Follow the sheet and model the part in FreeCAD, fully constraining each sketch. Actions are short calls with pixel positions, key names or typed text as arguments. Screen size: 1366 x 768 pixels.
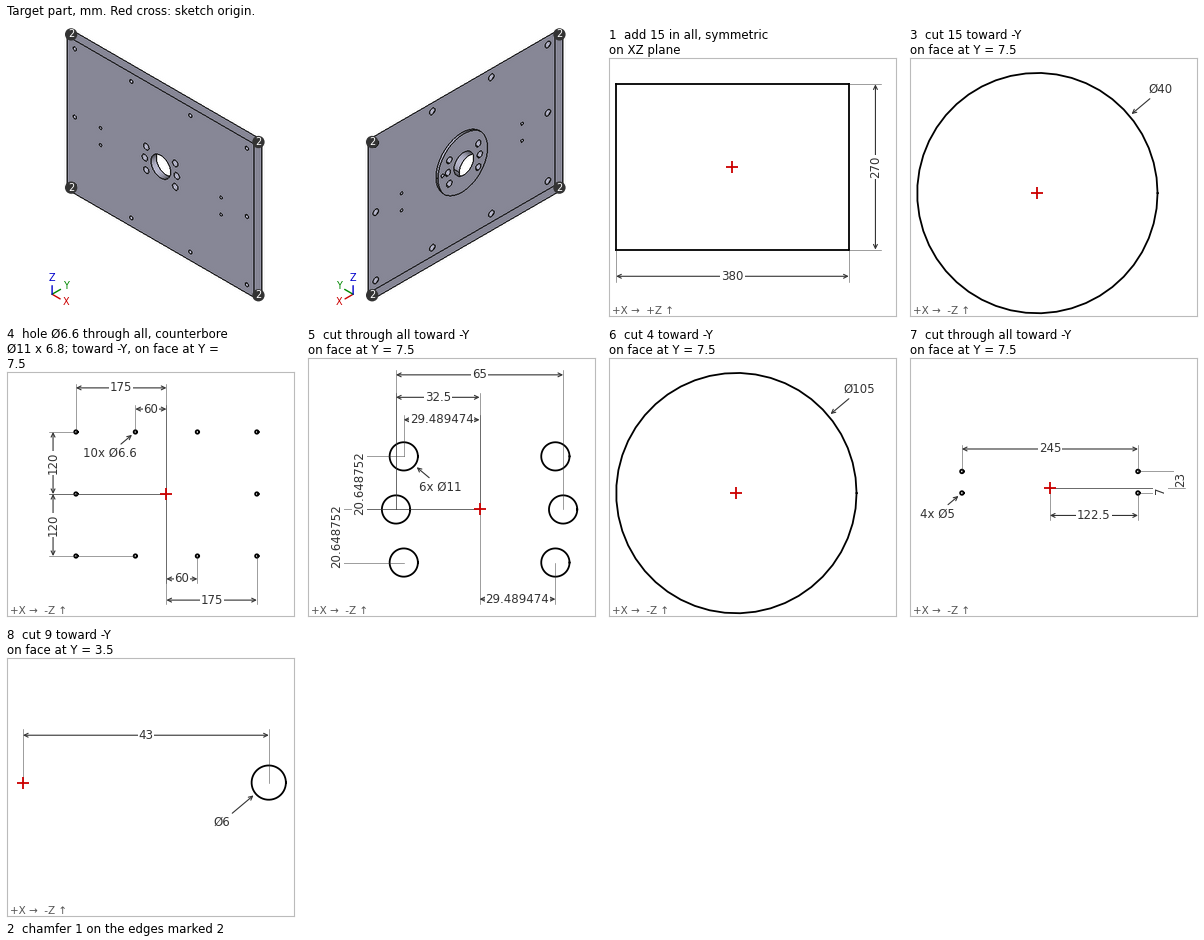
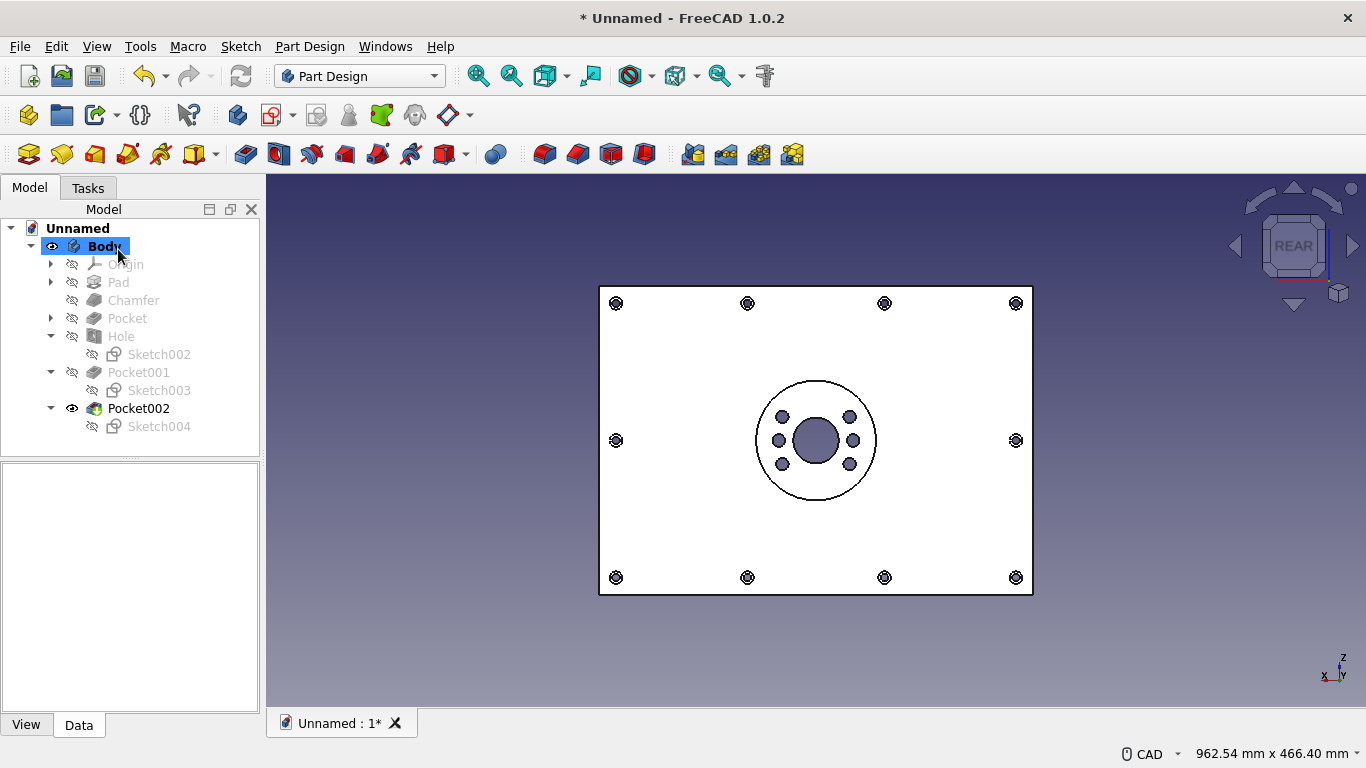
click(940, 395)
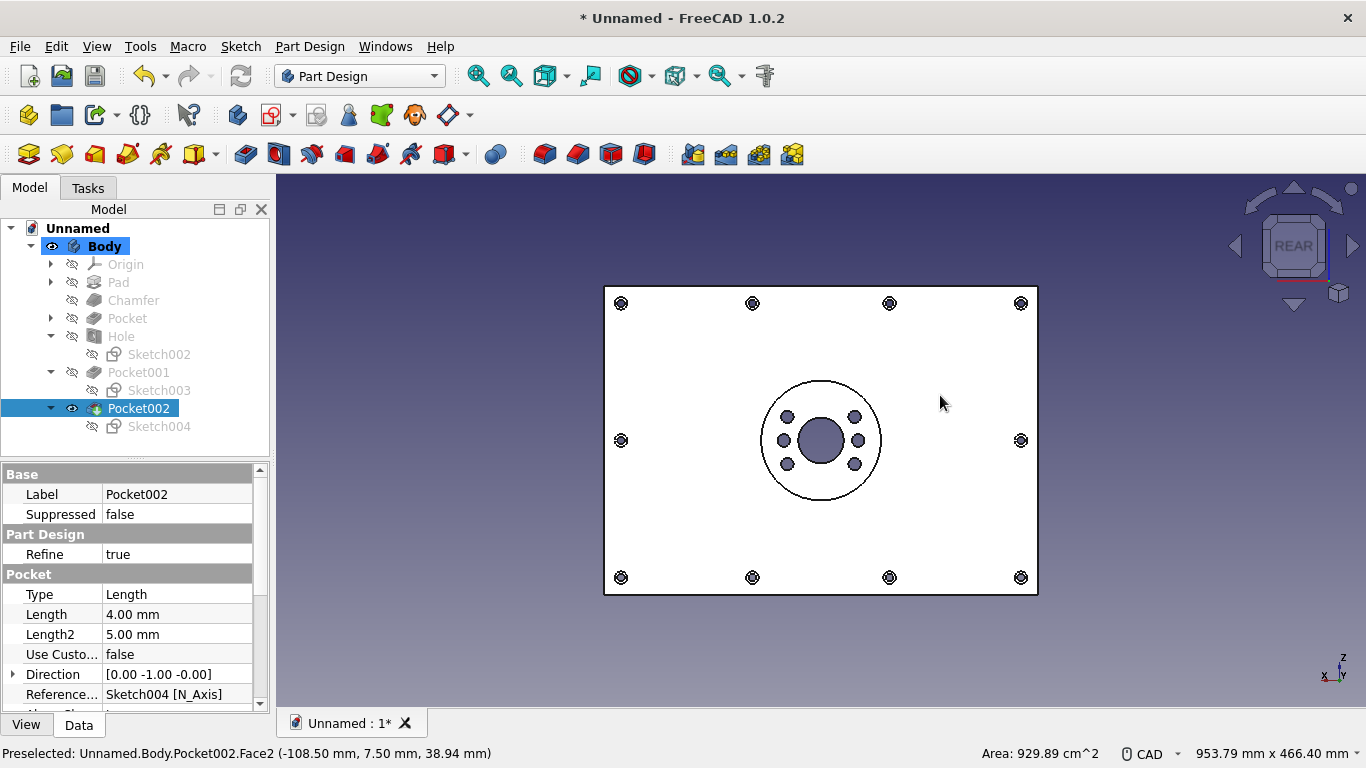
click(270, 116)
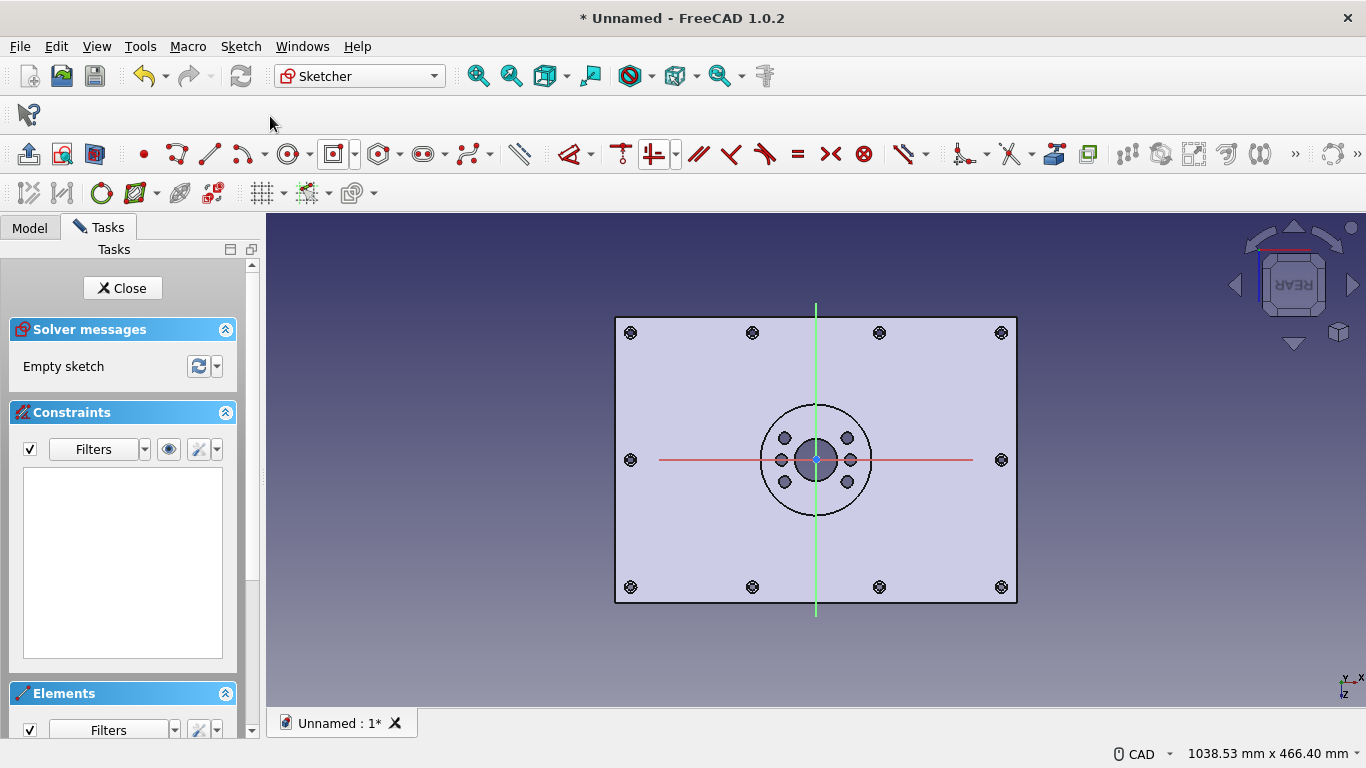
scroll(872, 445, up, 4)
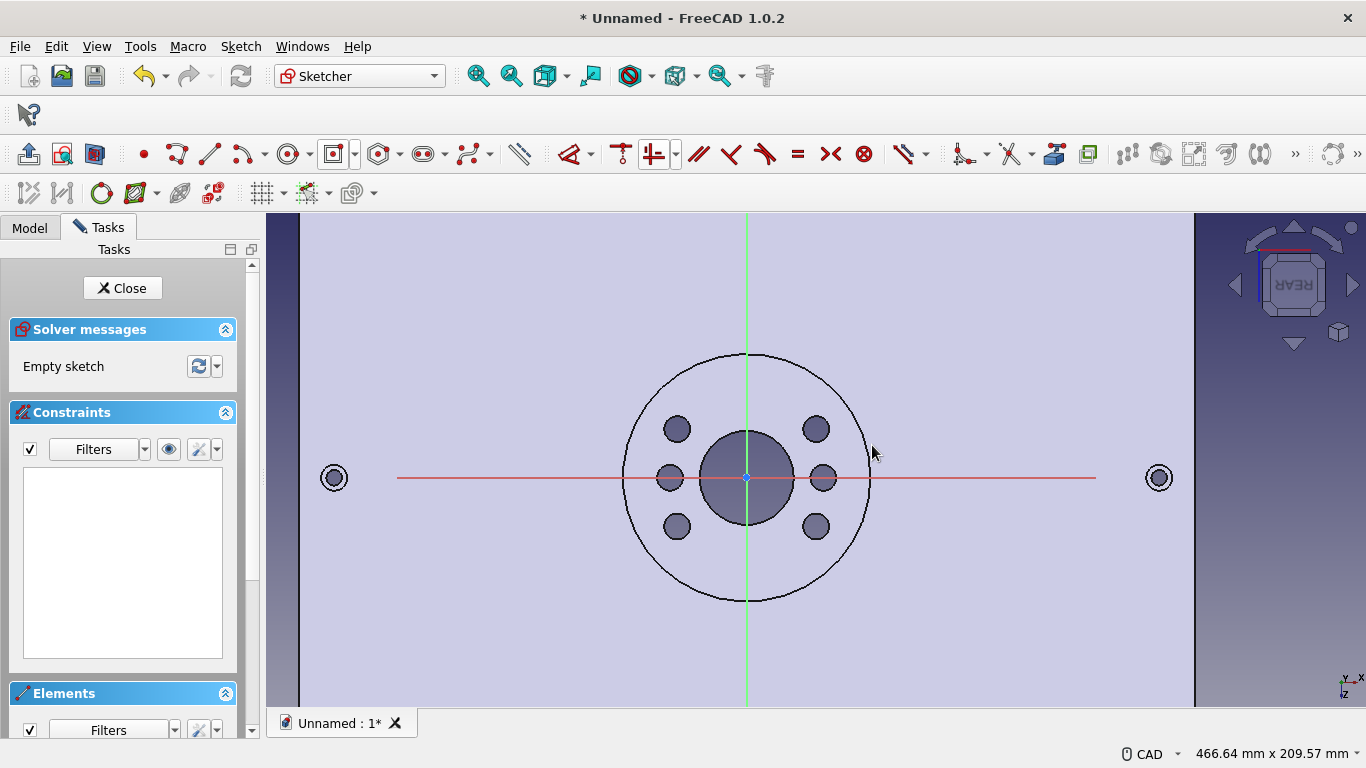
click(288, 154)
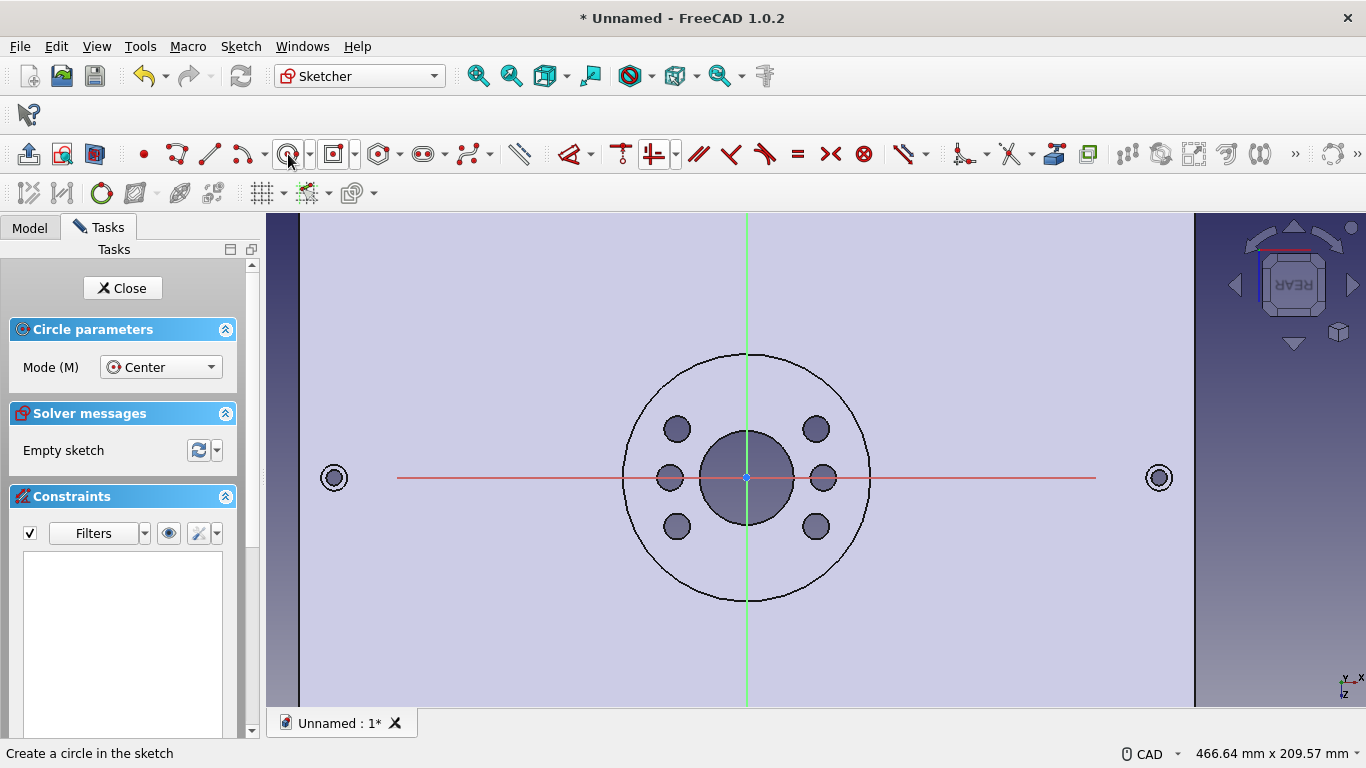
scroll(1035, 494, up, 7)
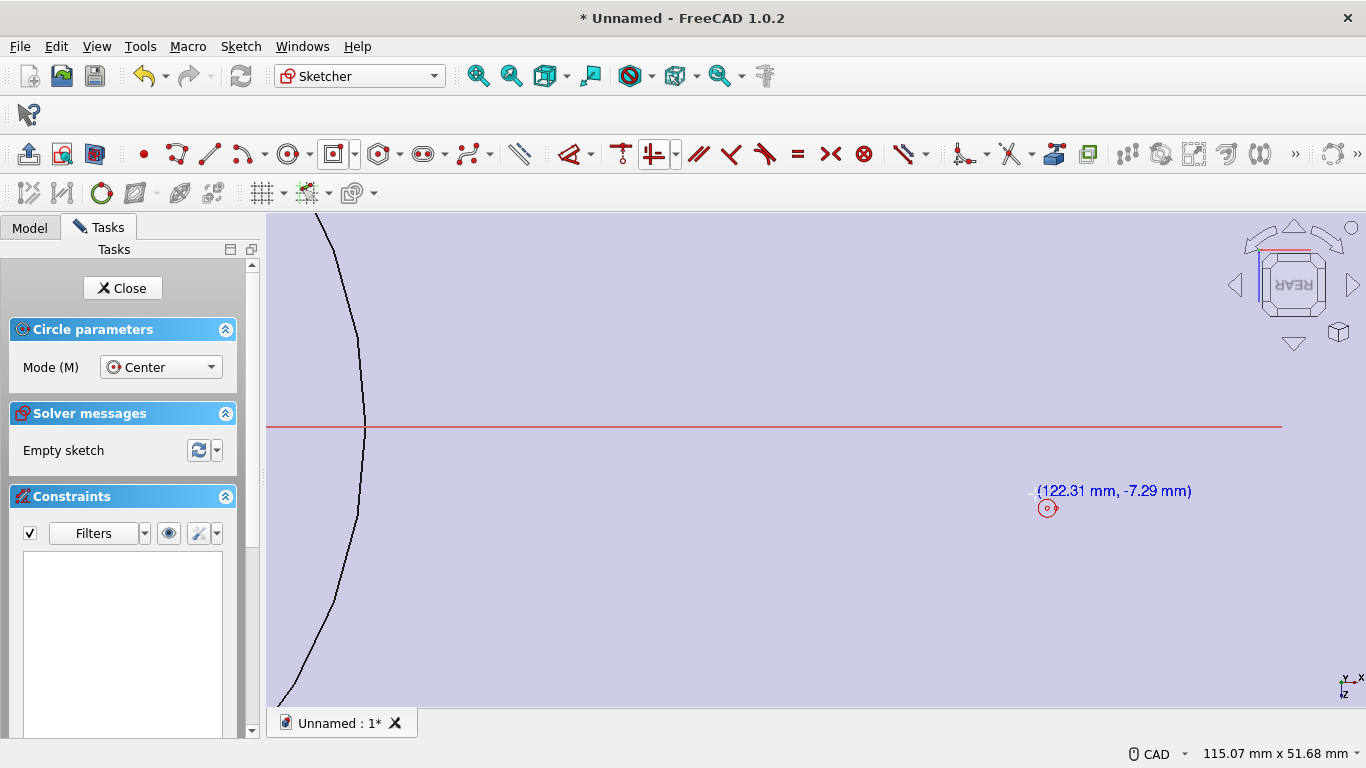
scroll(1037, 496, down, 7)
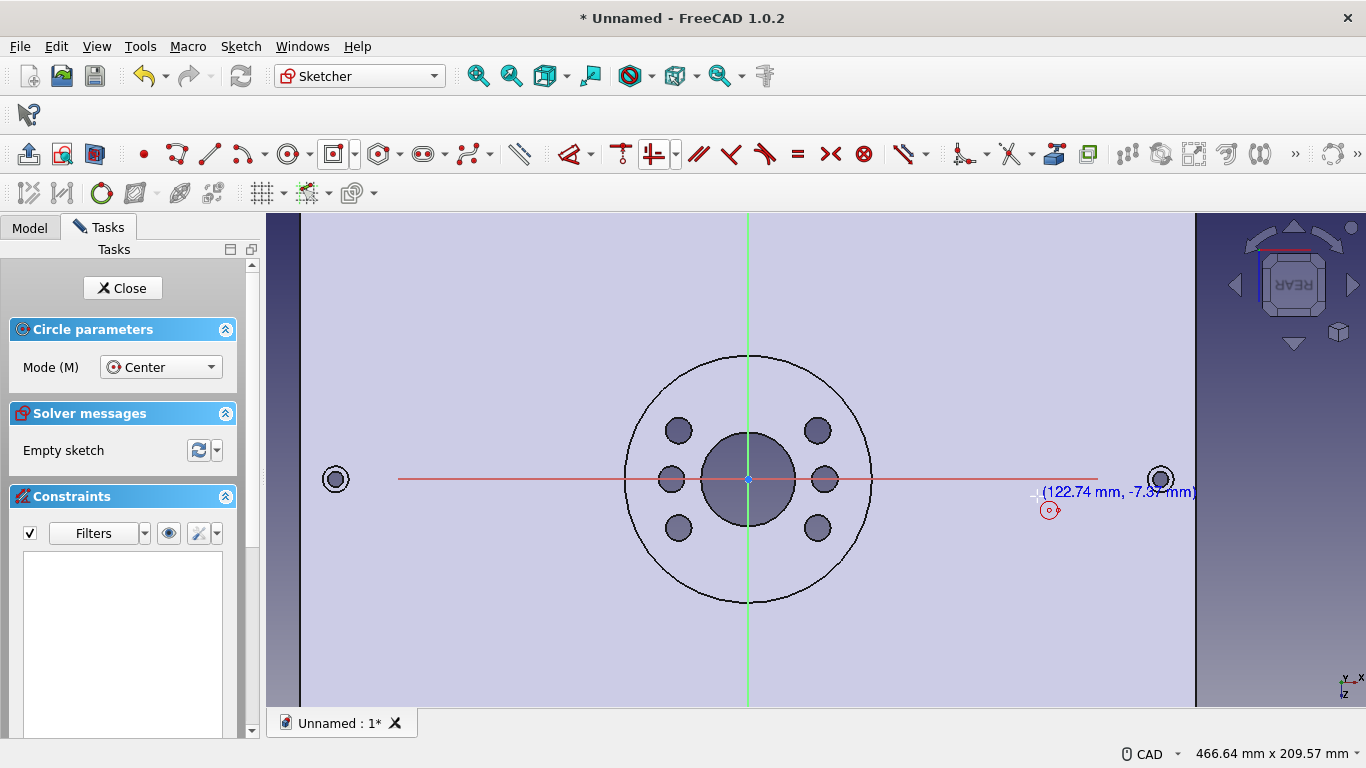
click(1037, 496)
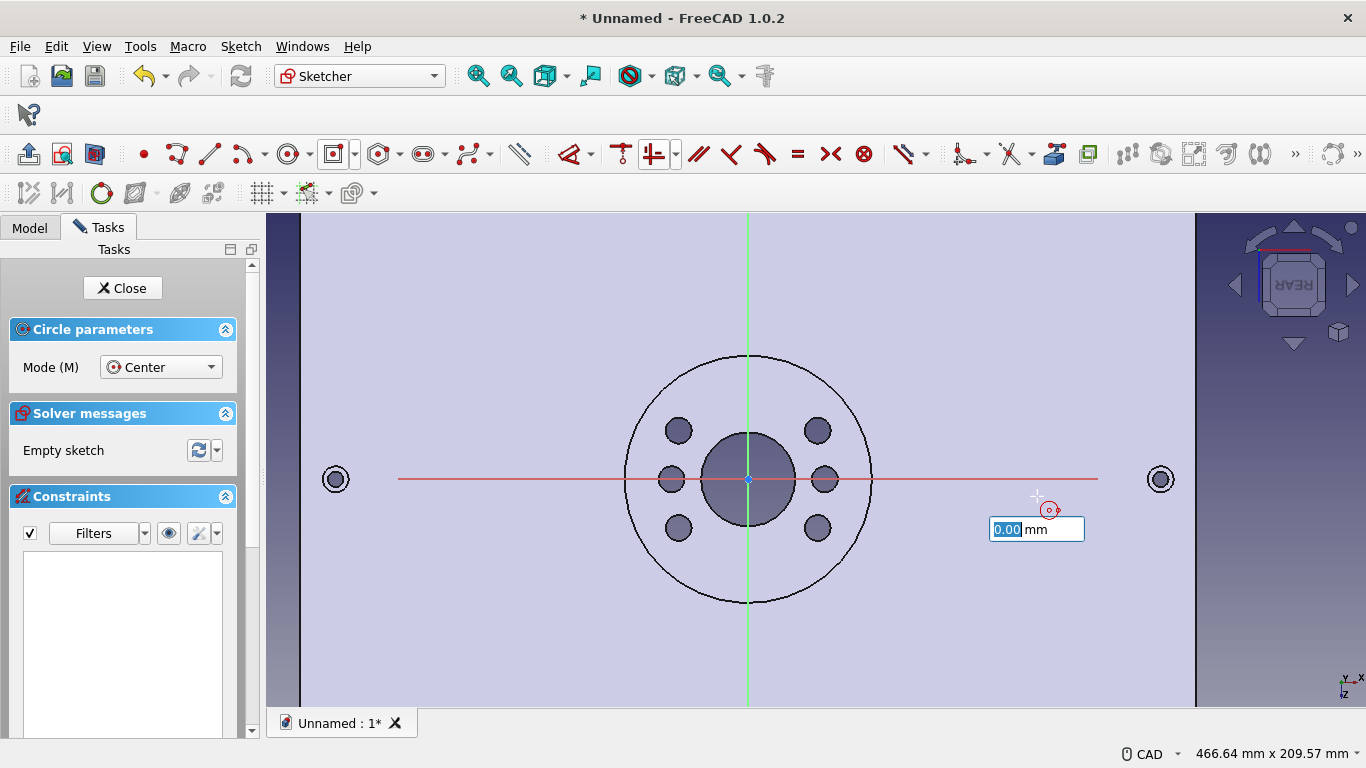
scroll(1041, 500, up, 5)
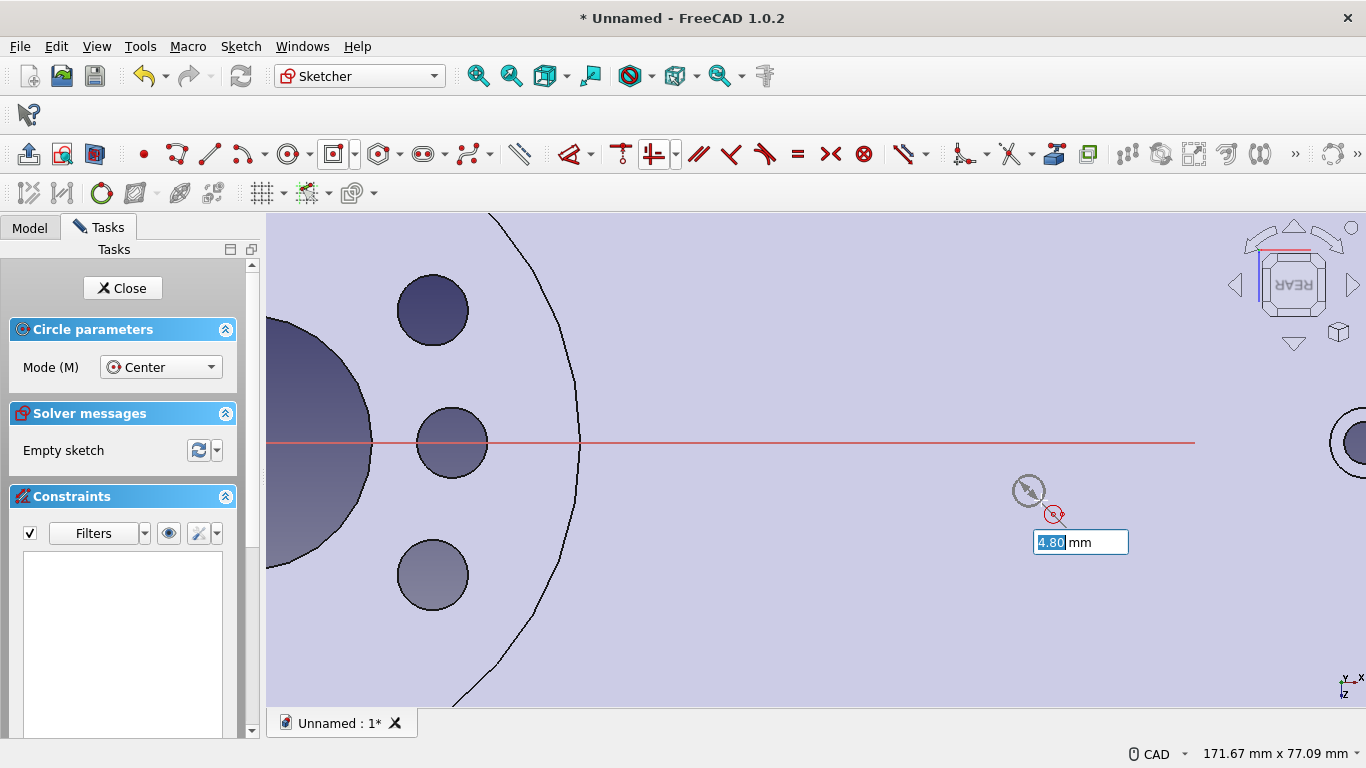
click(1040, 499)